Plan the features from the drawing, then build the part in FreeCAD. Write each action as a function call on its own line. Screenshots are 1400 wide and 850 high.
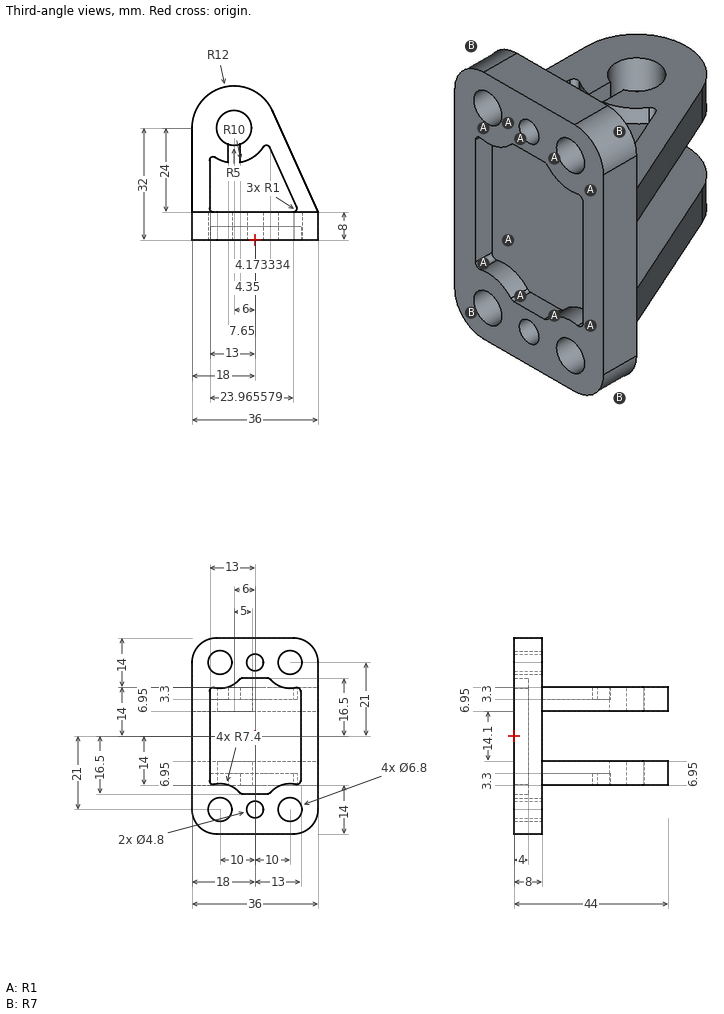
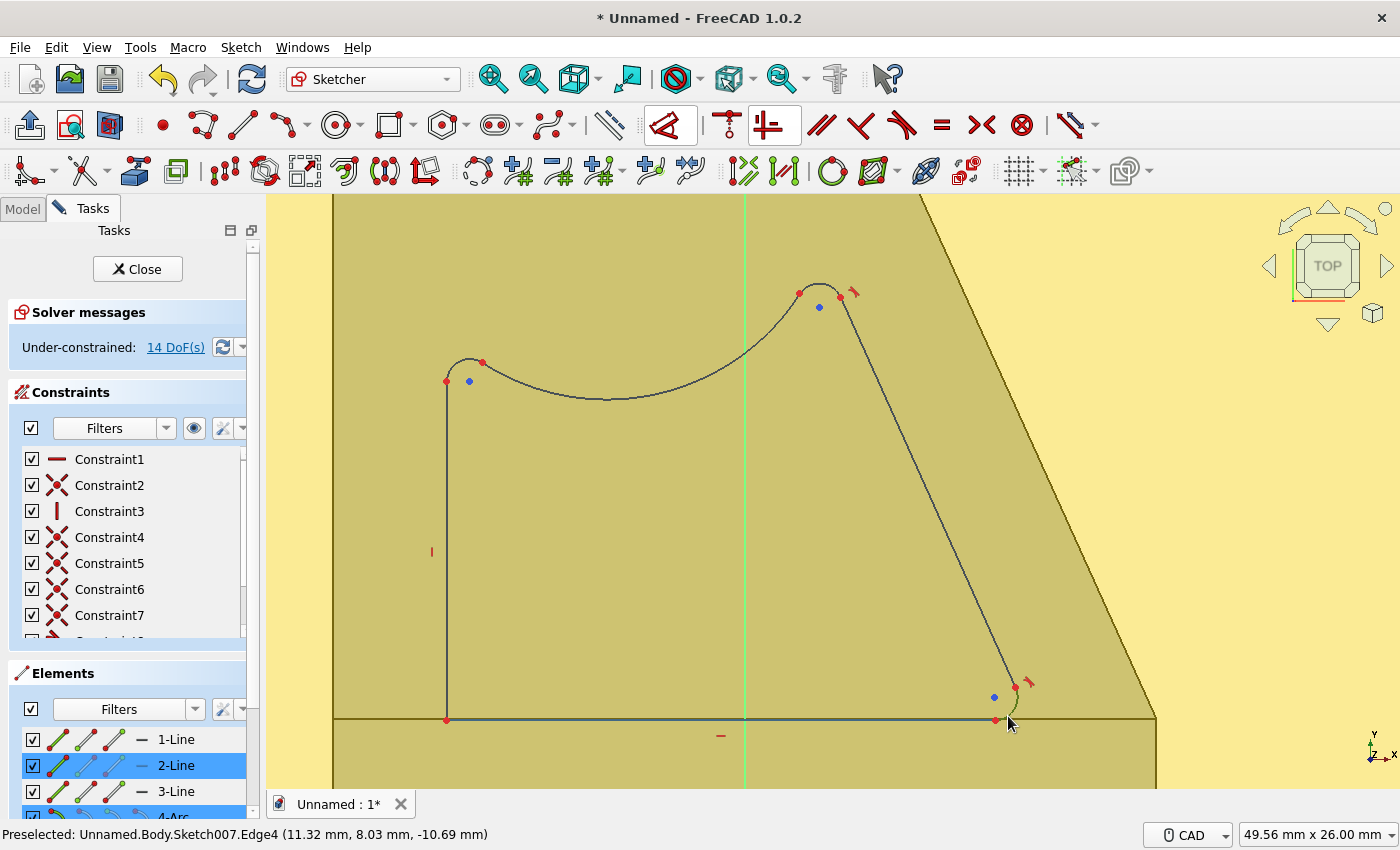
key(t)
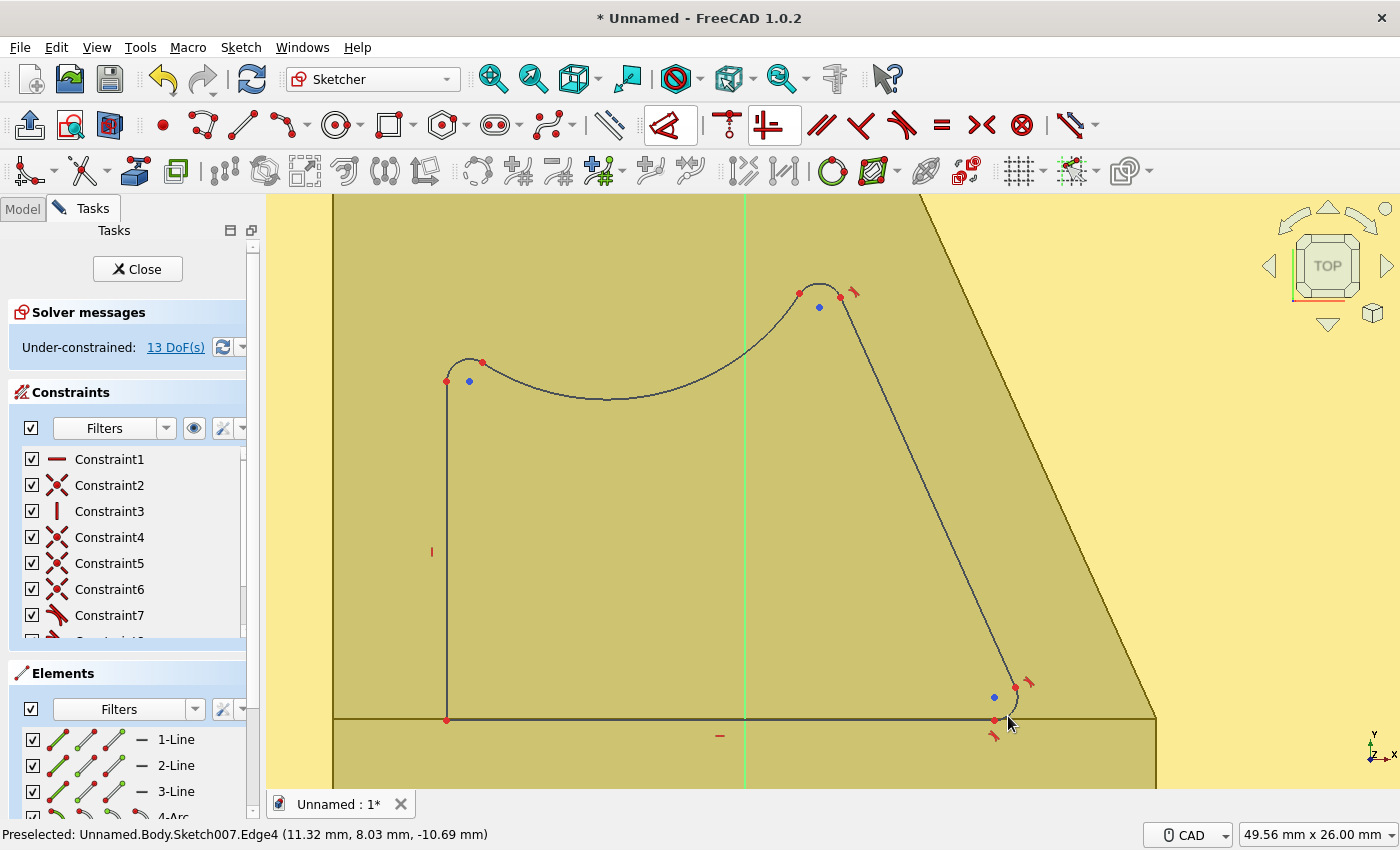
click(447, 619)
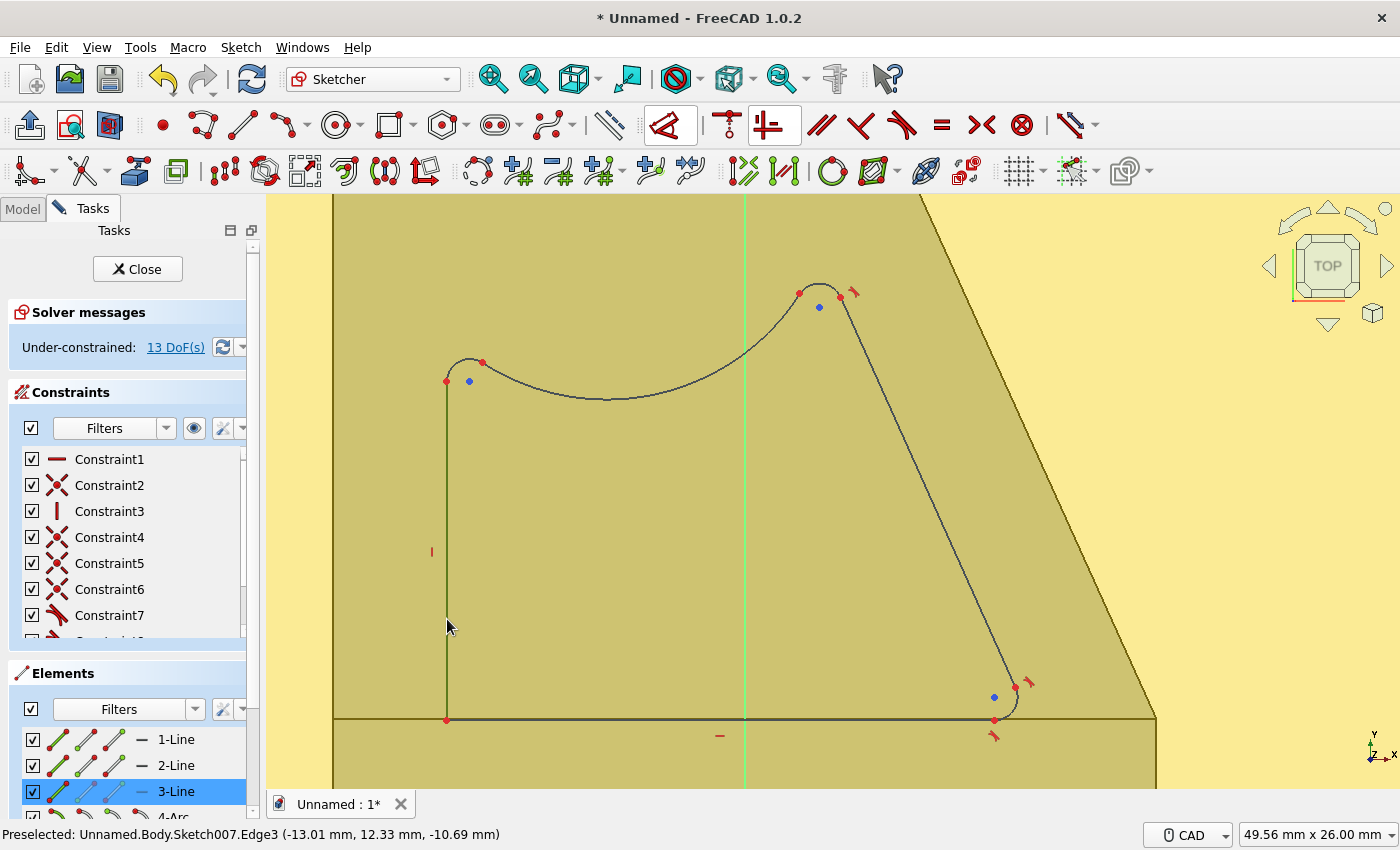
click(468, 359)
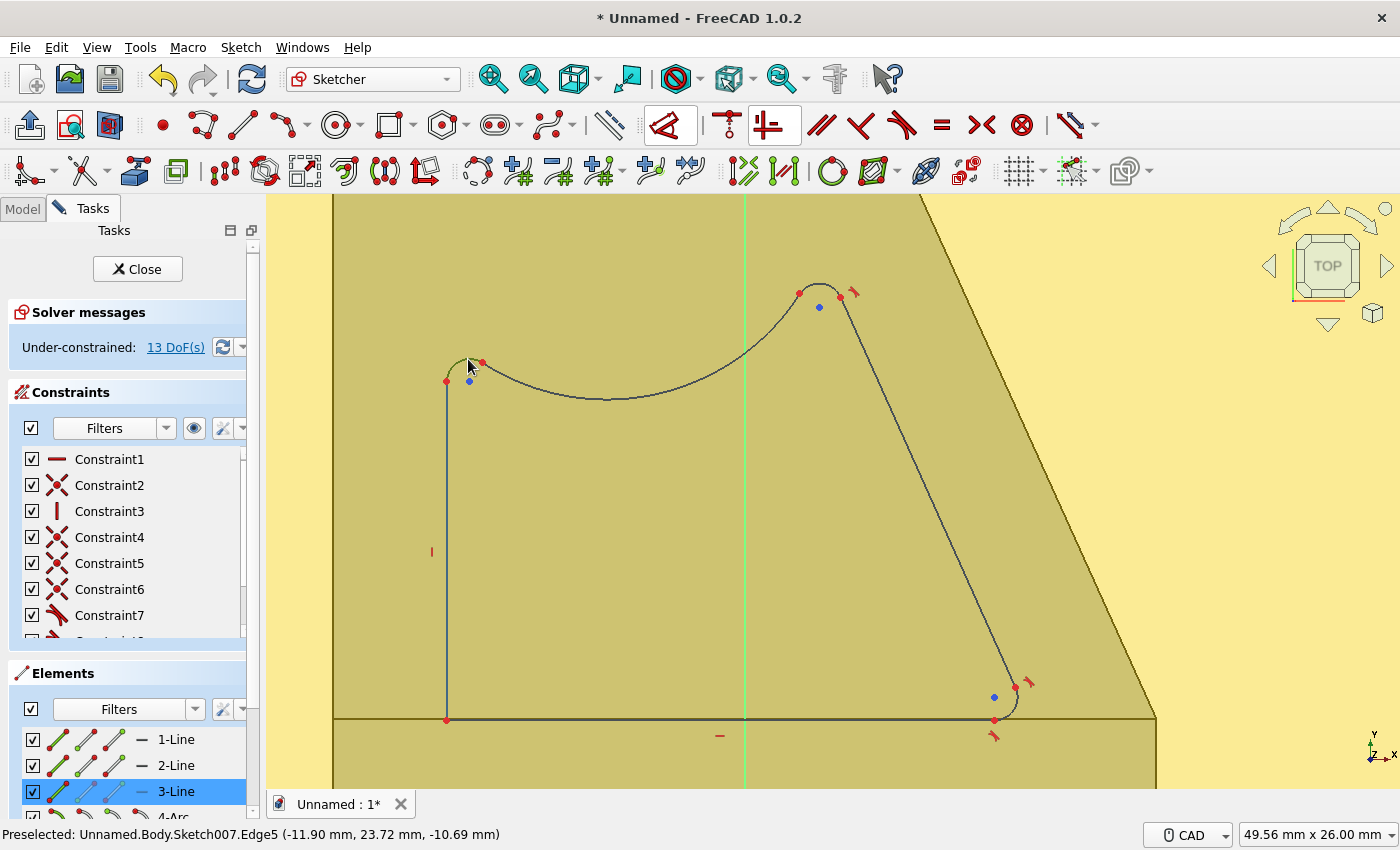
click(902, 126)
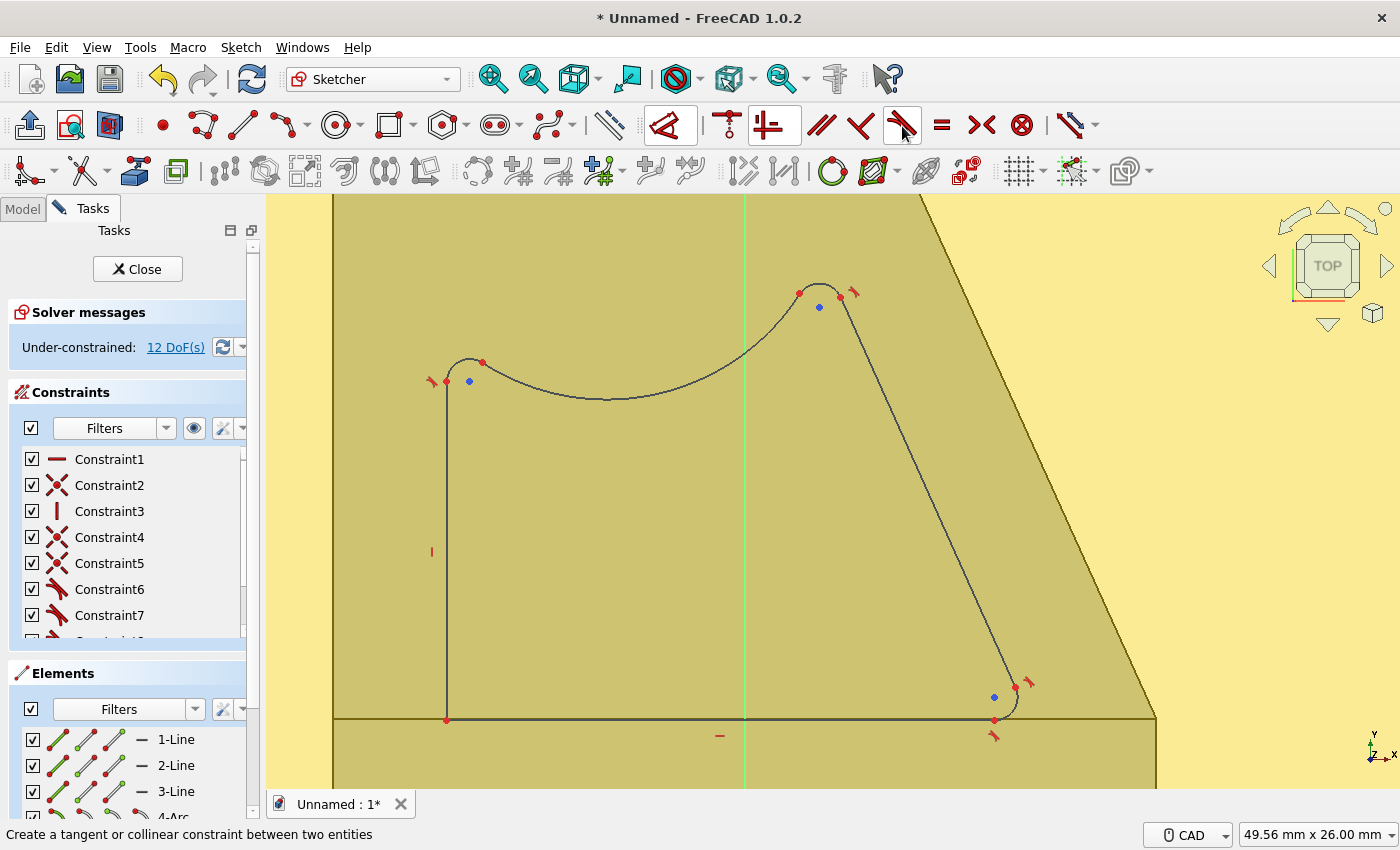
click(468, 359)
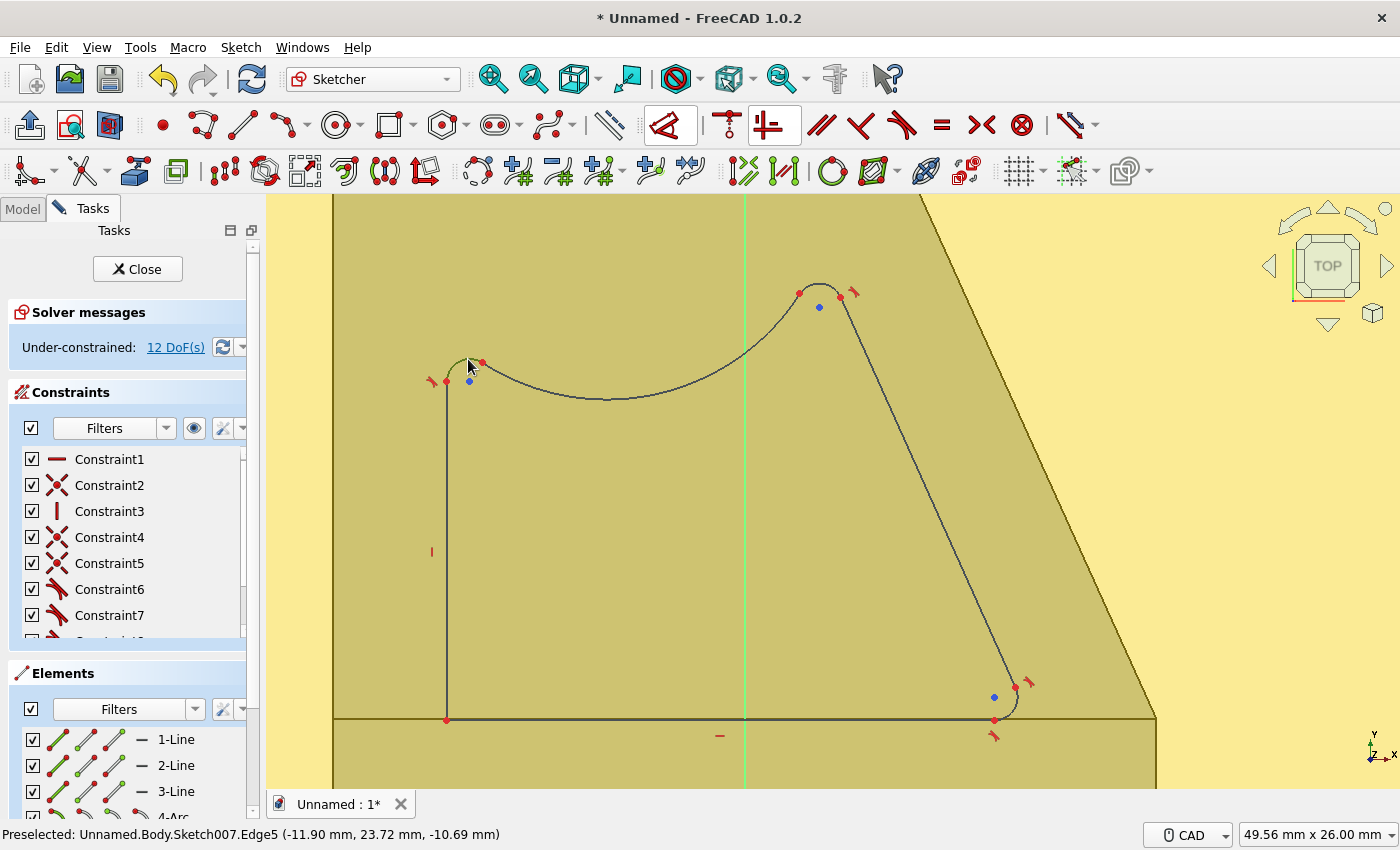
click(584, 398)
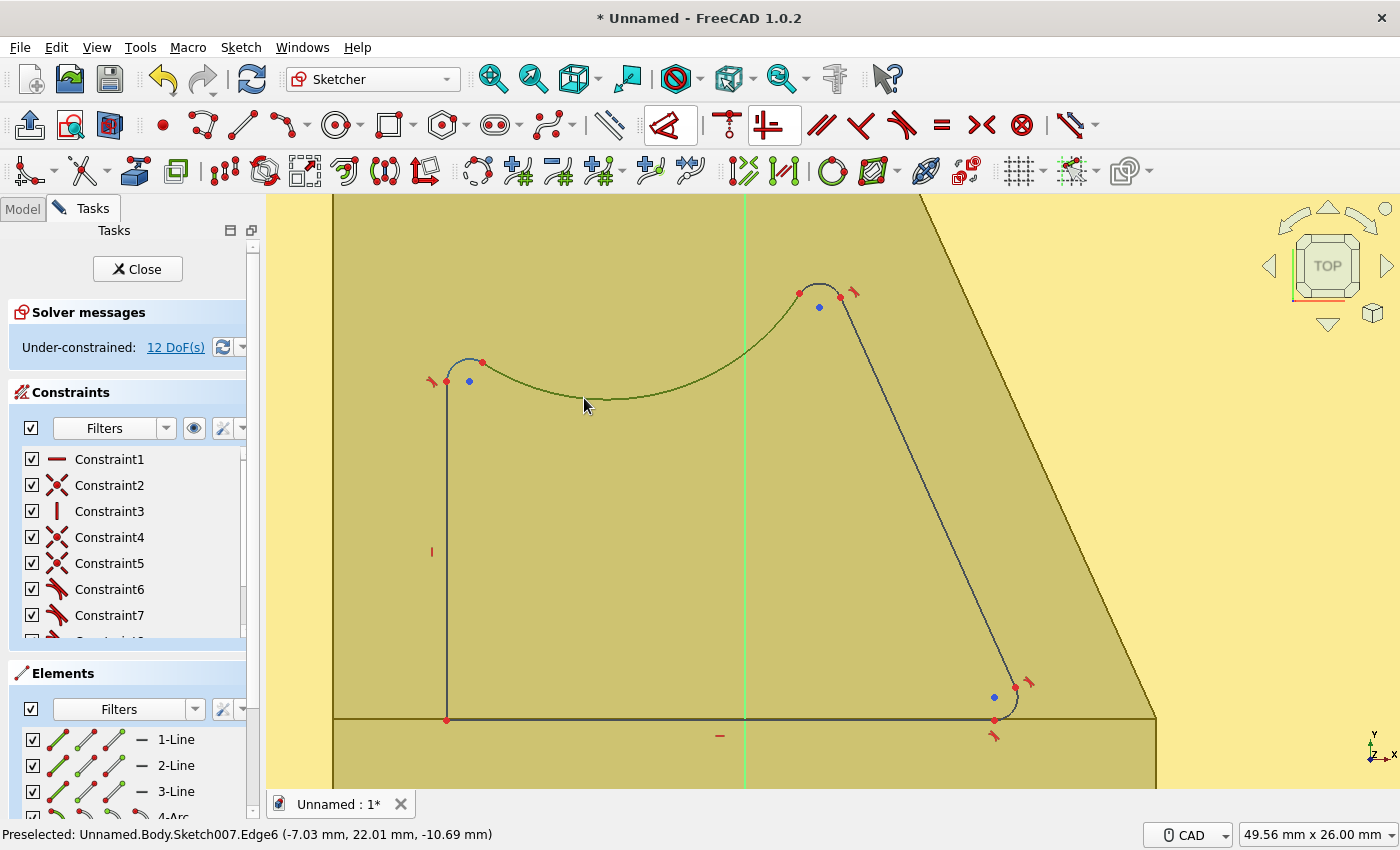
click(902, 126)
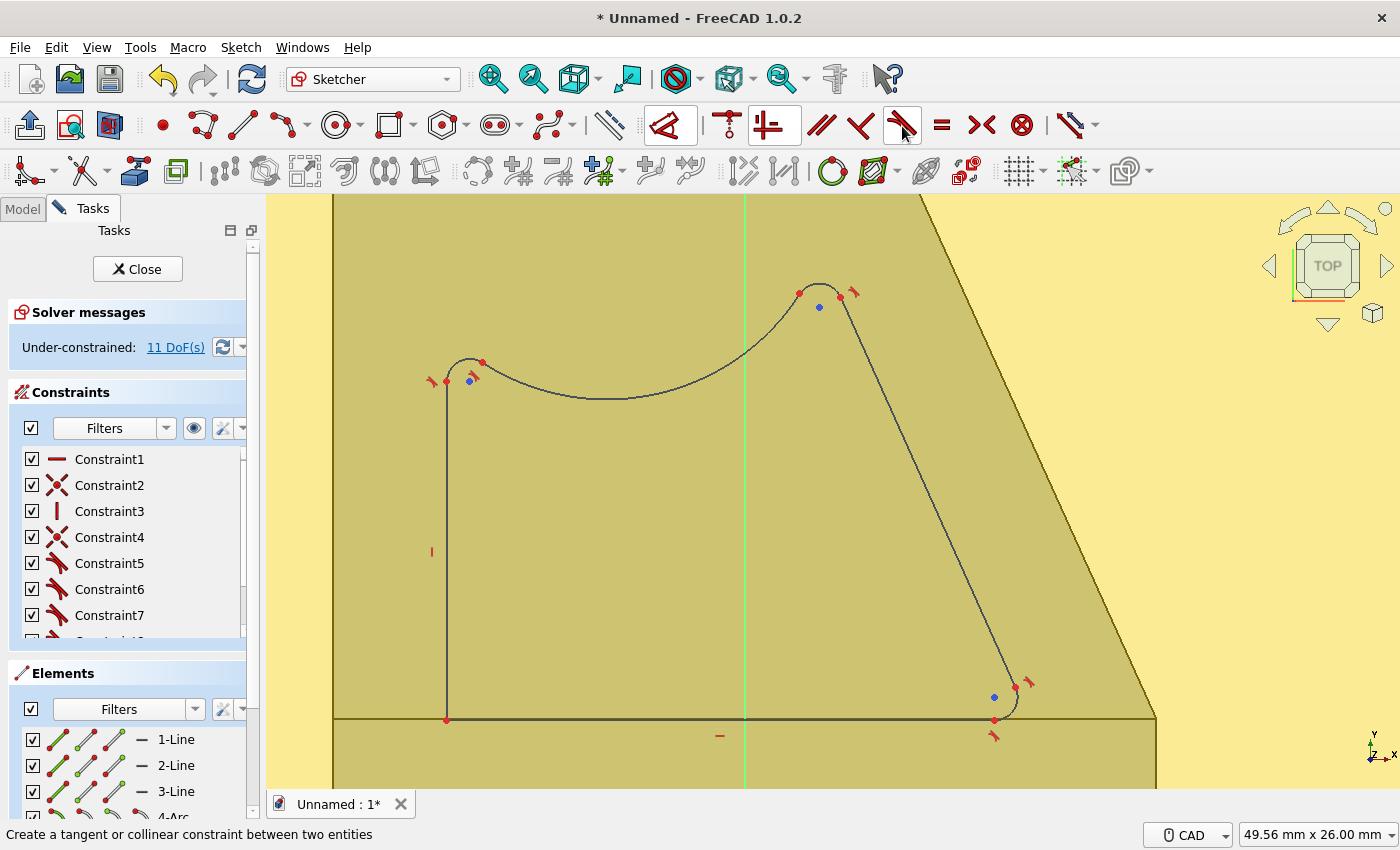
click(584, 398)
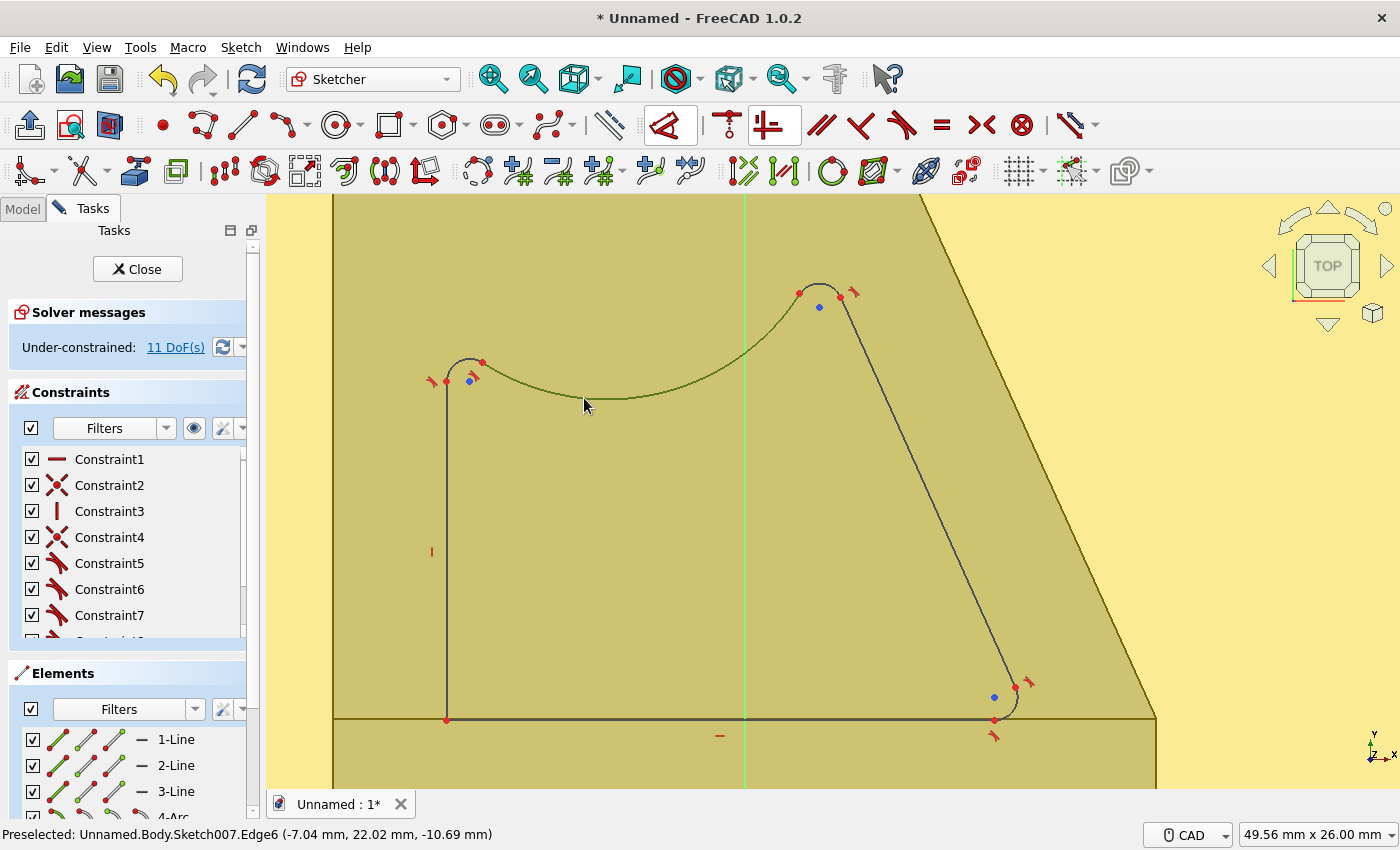
click(831, 287)